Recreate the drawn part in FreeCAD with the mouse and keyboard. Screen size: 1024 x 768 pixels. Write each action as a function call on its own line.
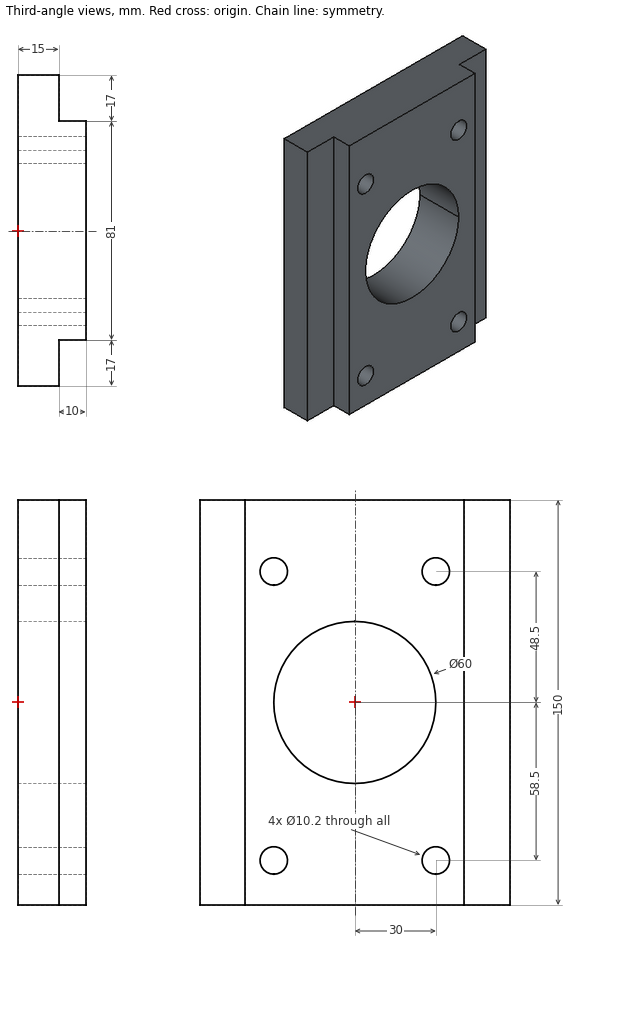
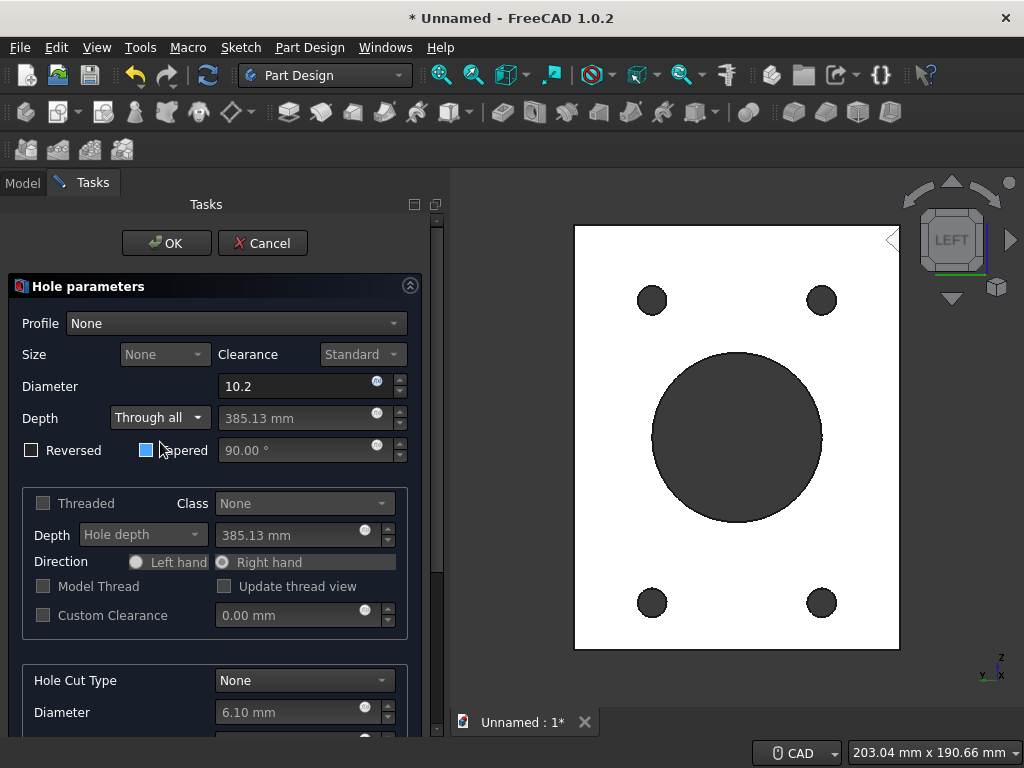
click(167, 243)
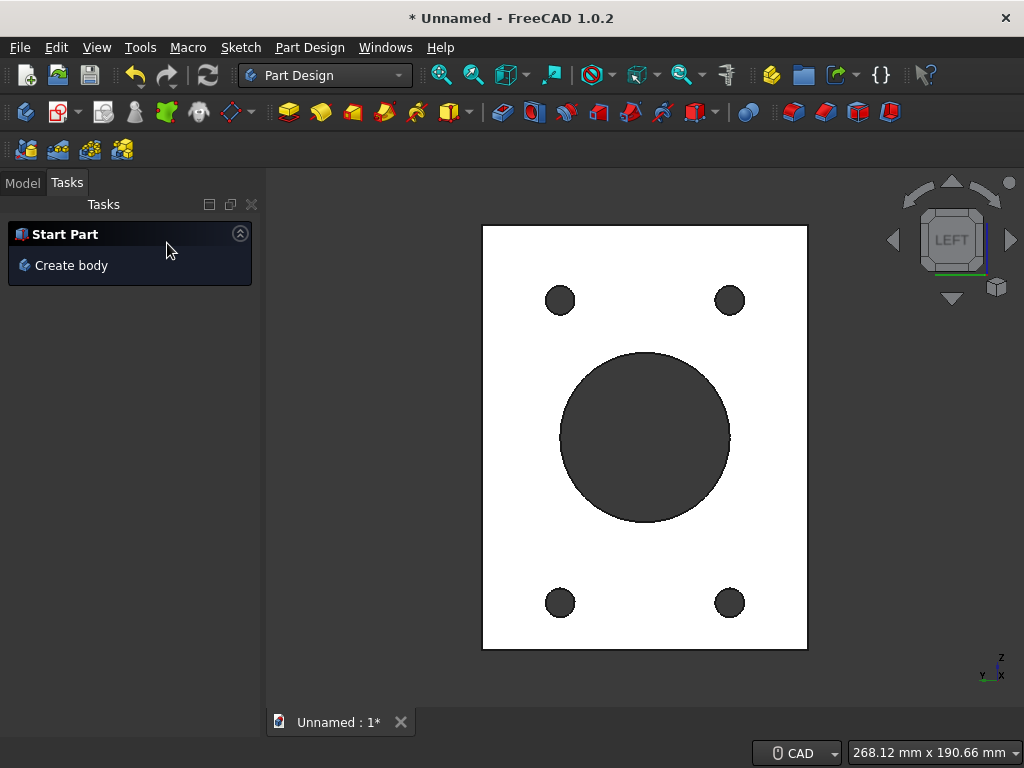
key(0)